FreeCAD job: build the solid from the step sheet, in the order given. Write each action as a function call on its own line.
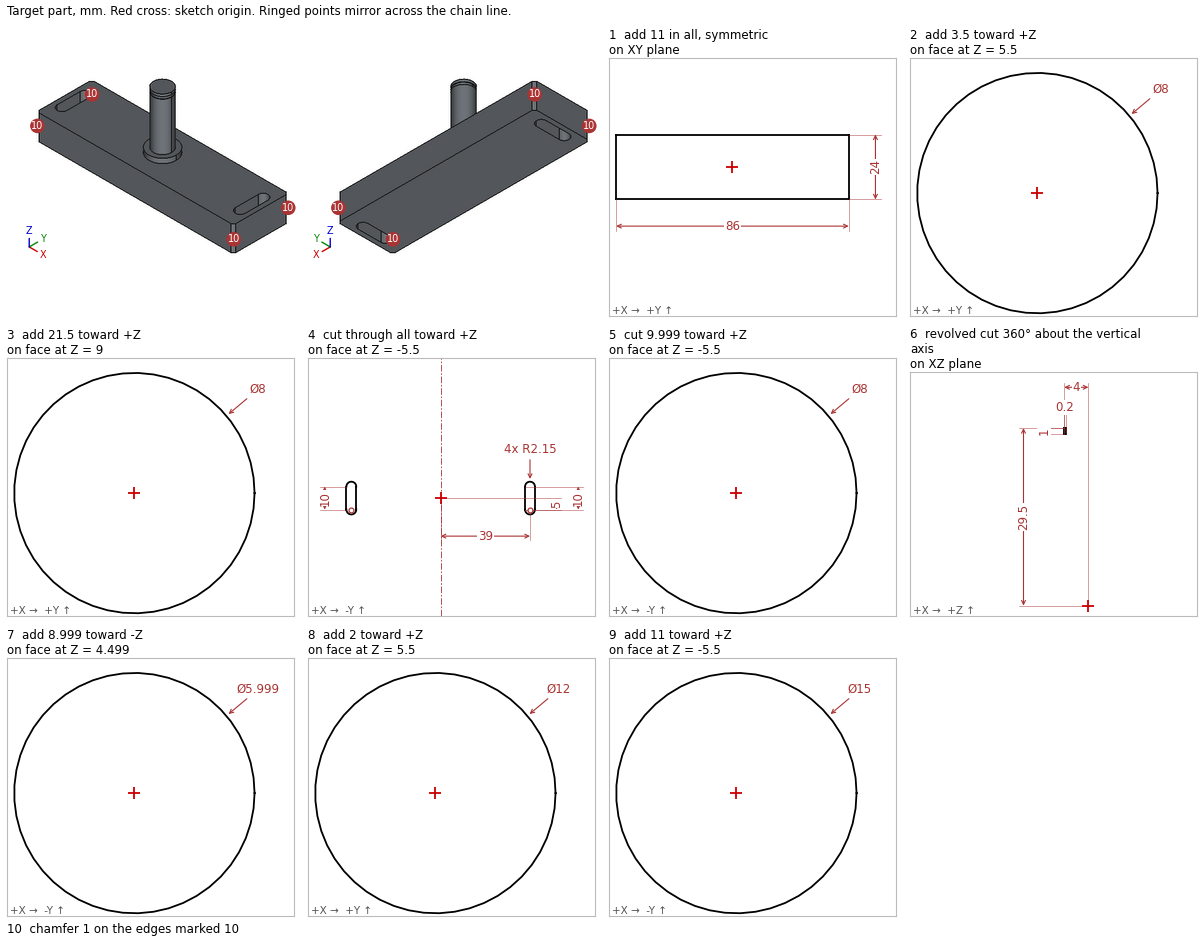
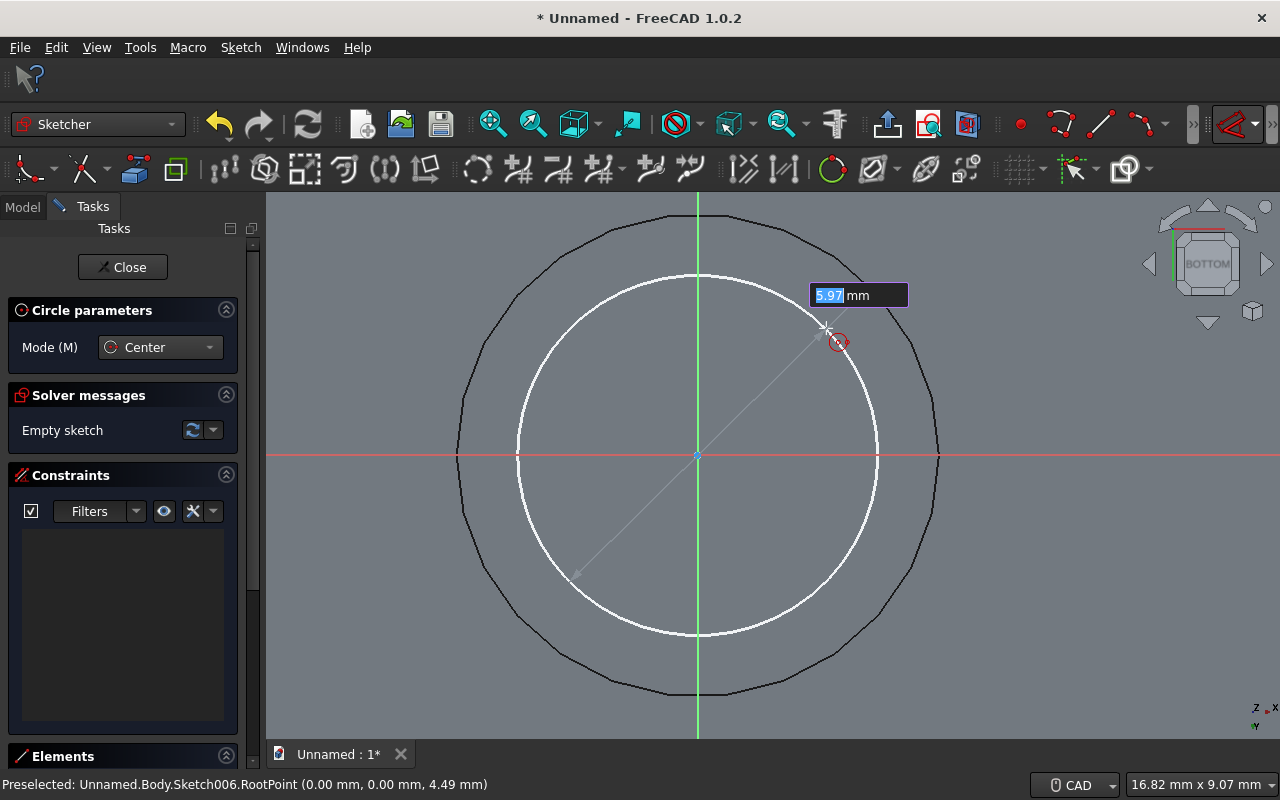
text(5.999)
key(Return)
key(Escape)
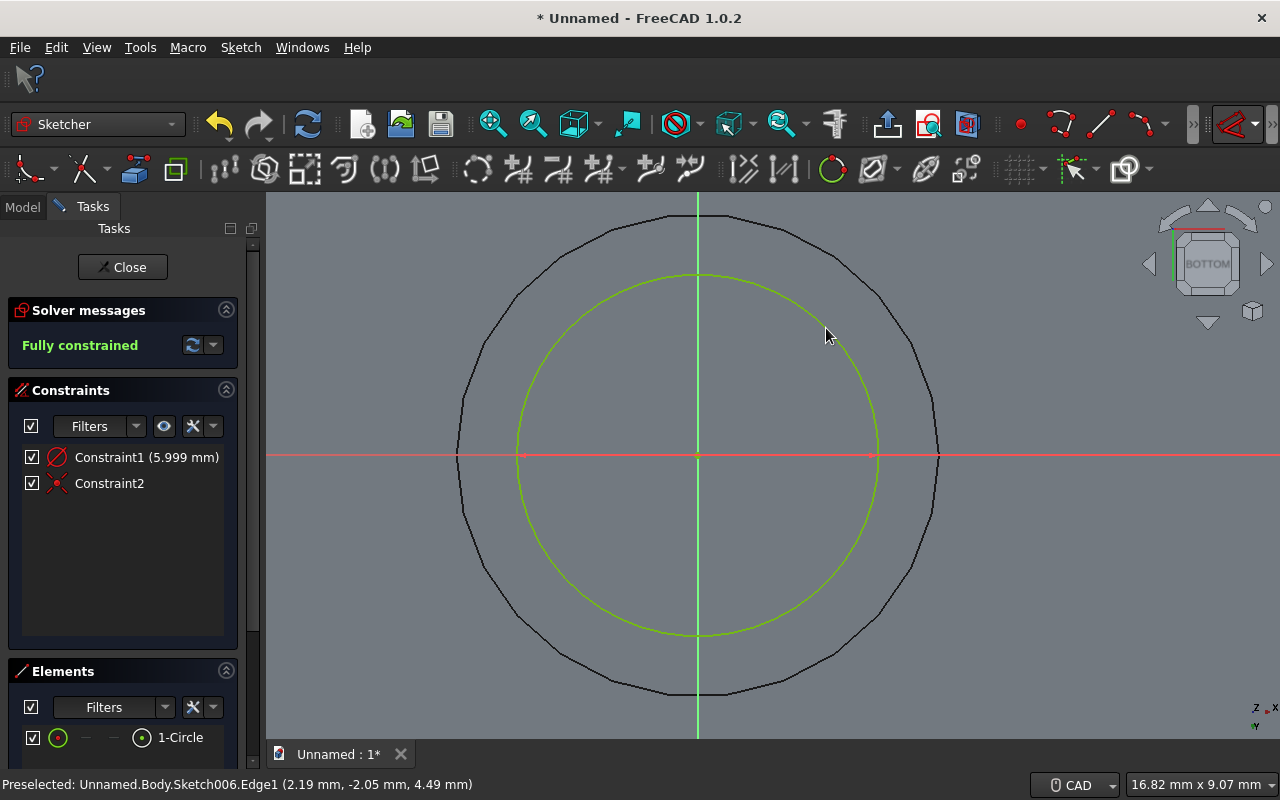
click(123, 267)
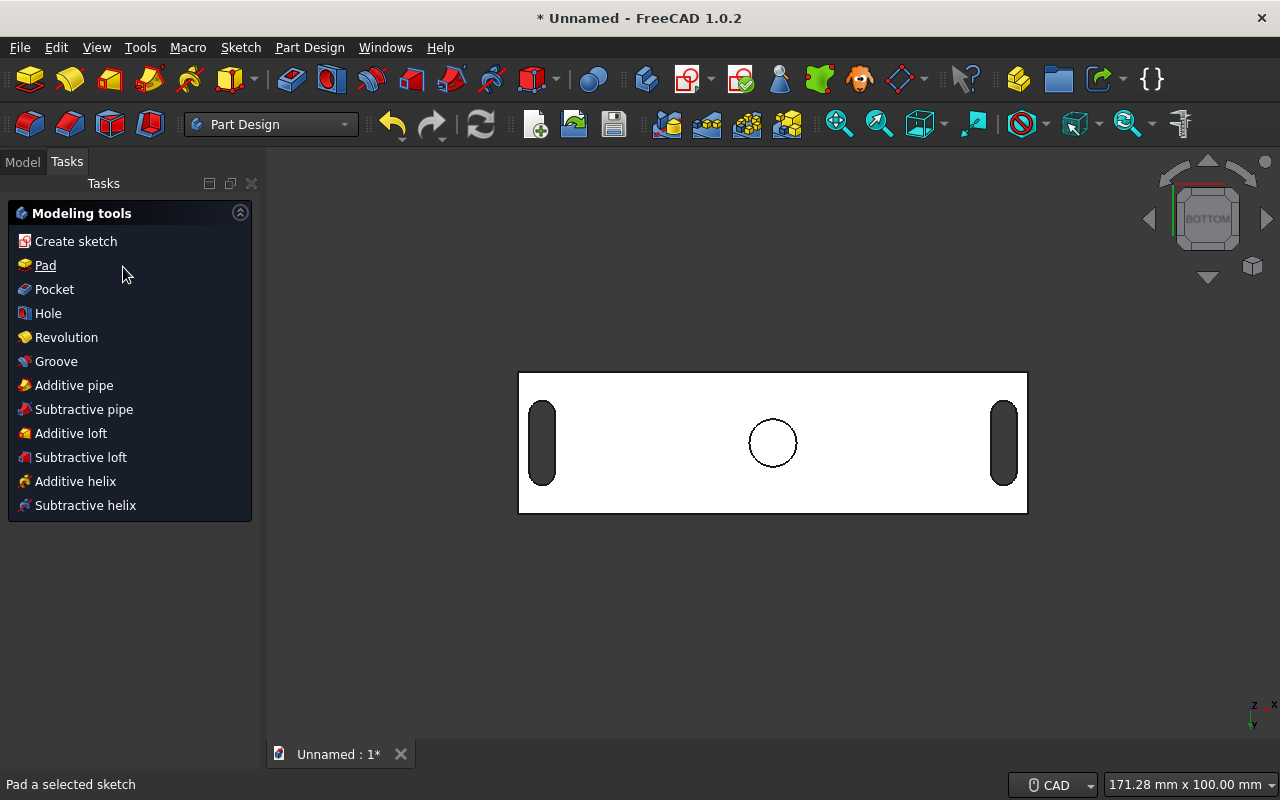
click(30, 80)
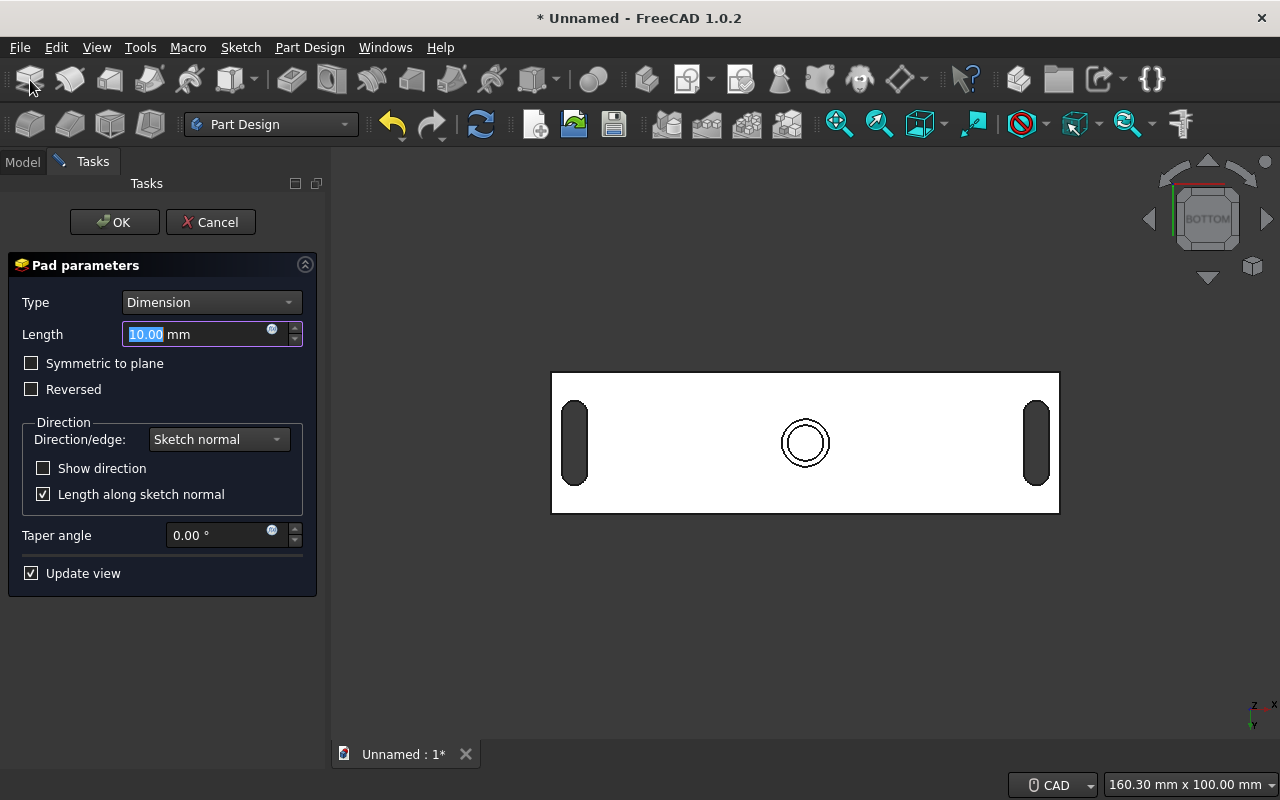
text(8.999)
key(Tab)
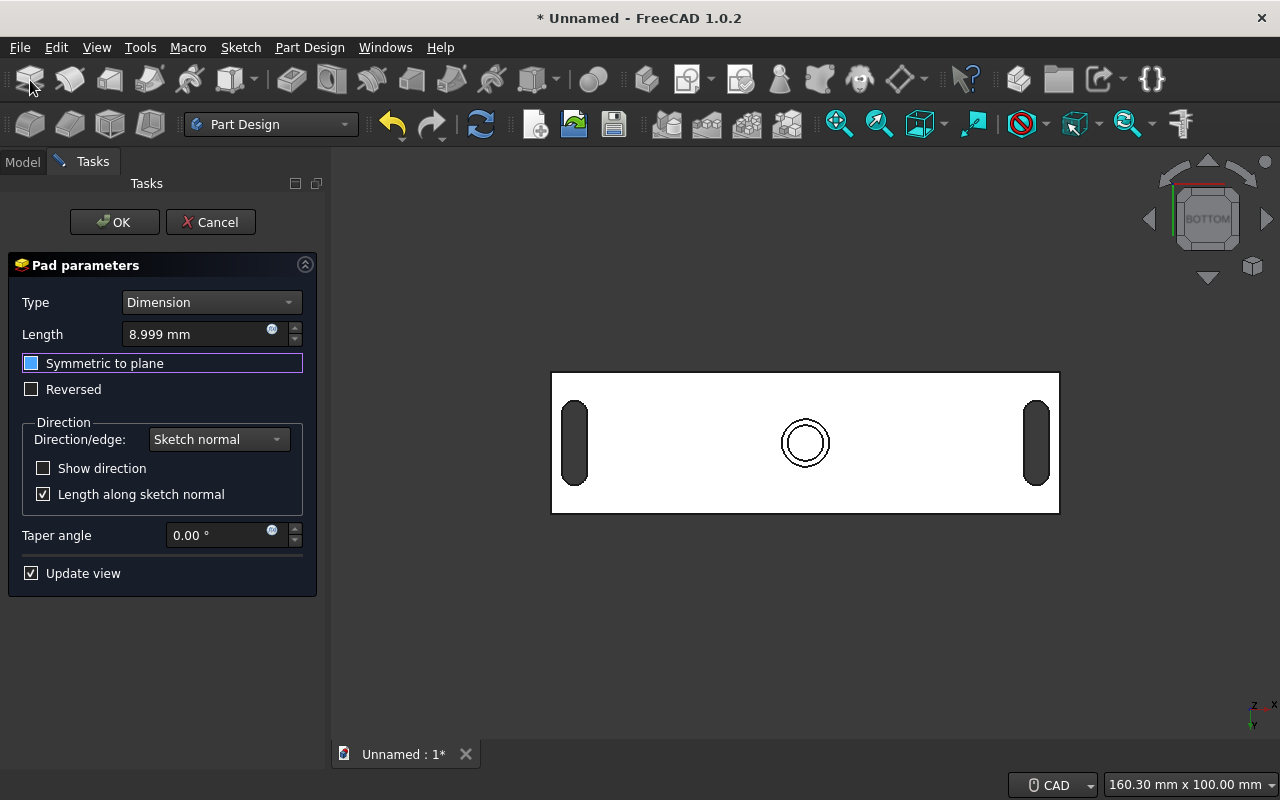
click(115, 222)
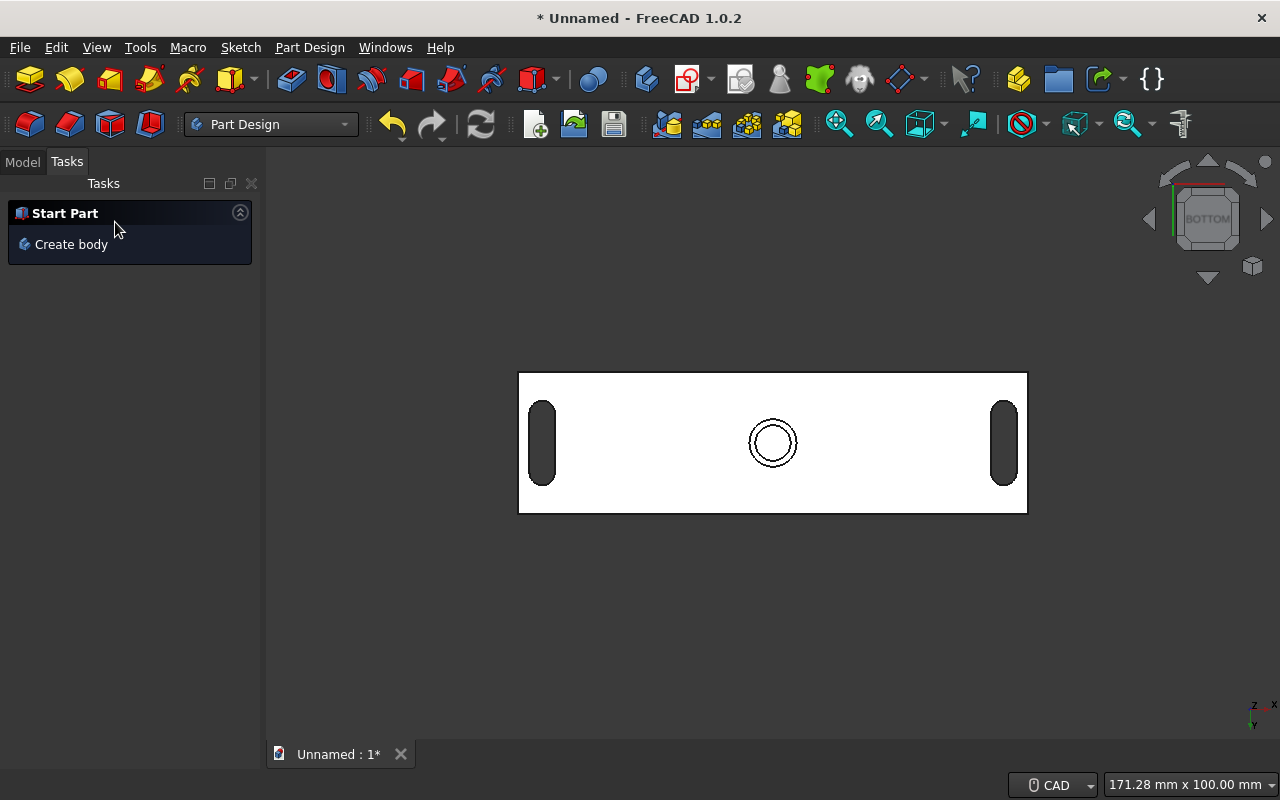
key(0)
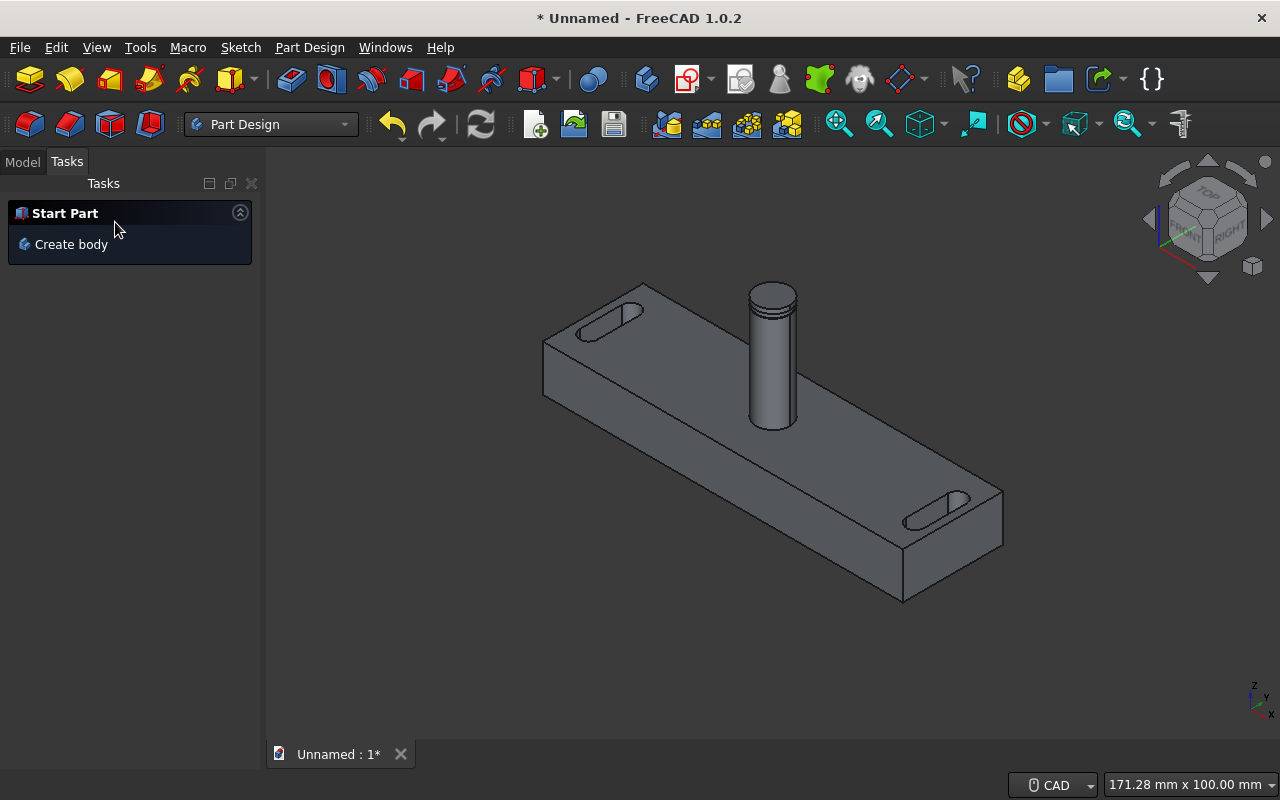
click(876, 475)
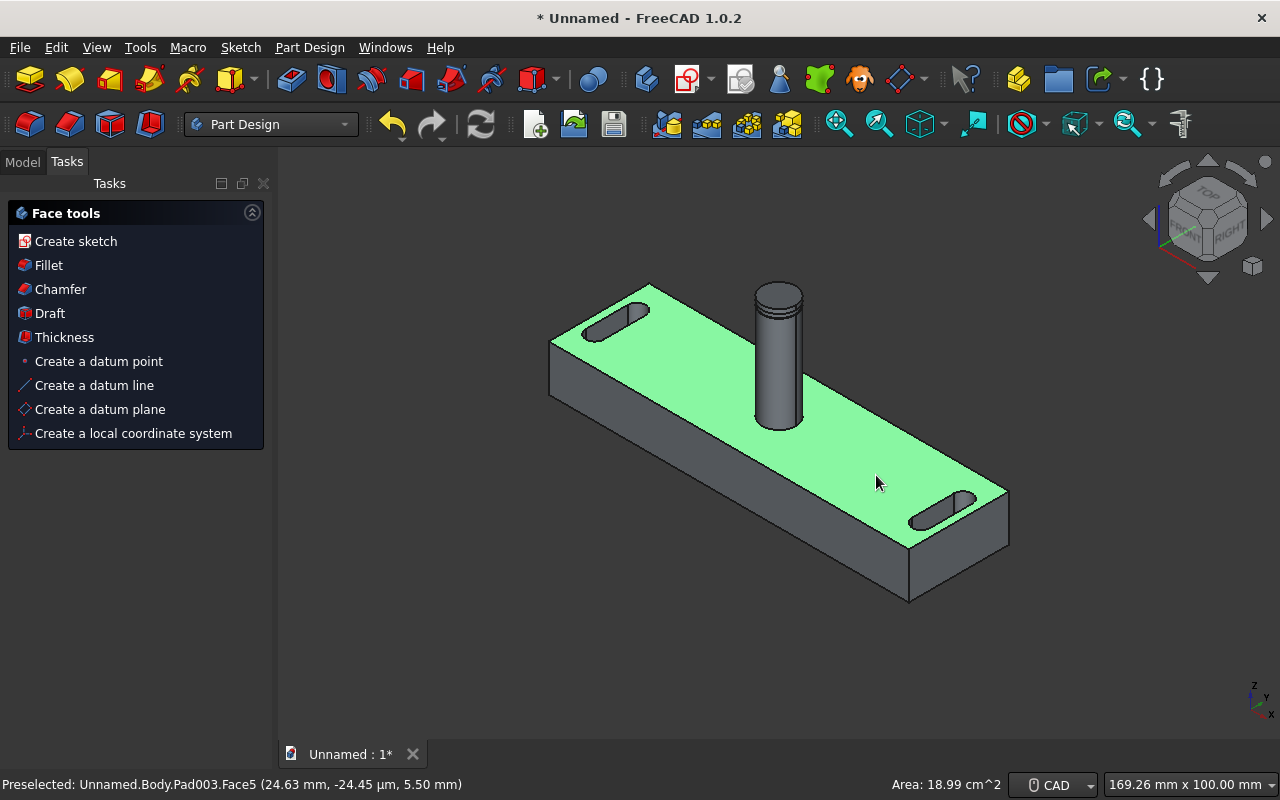
click(688, 80)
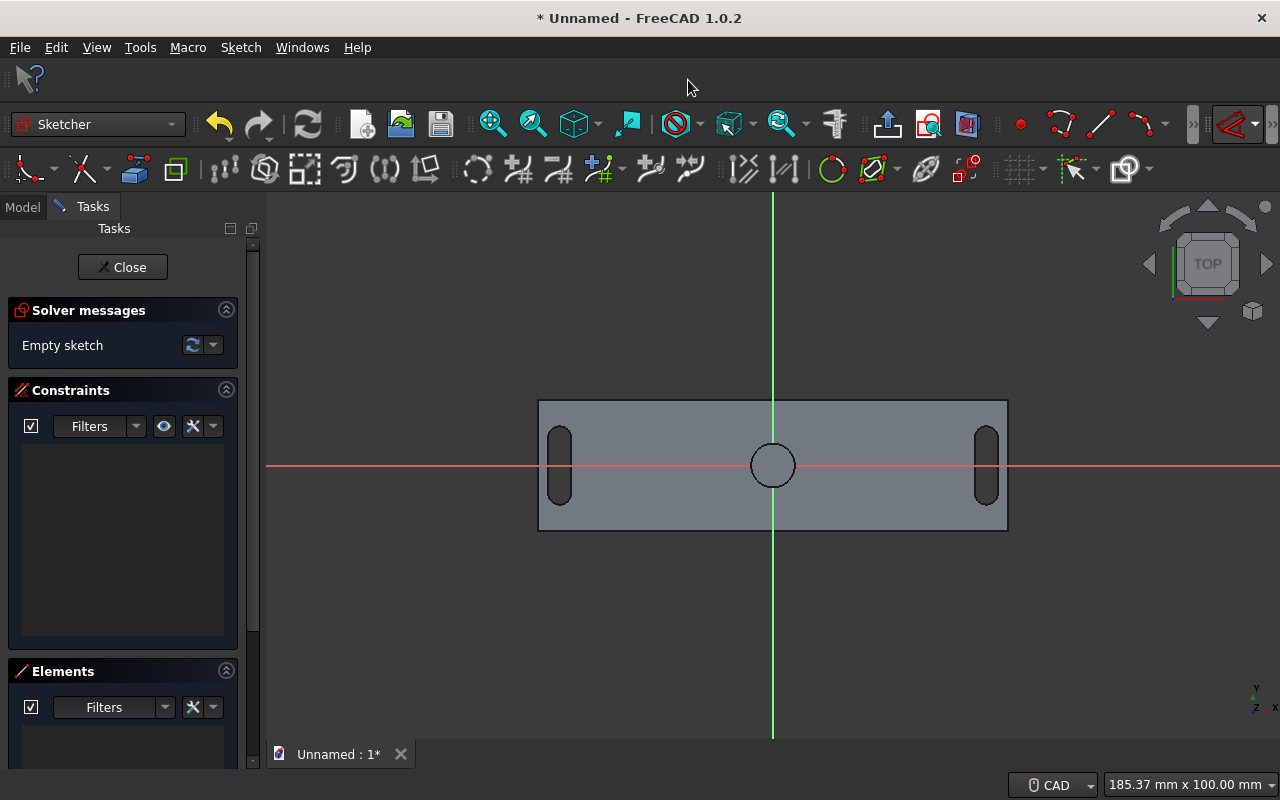
scroll(790, 465, up, 8)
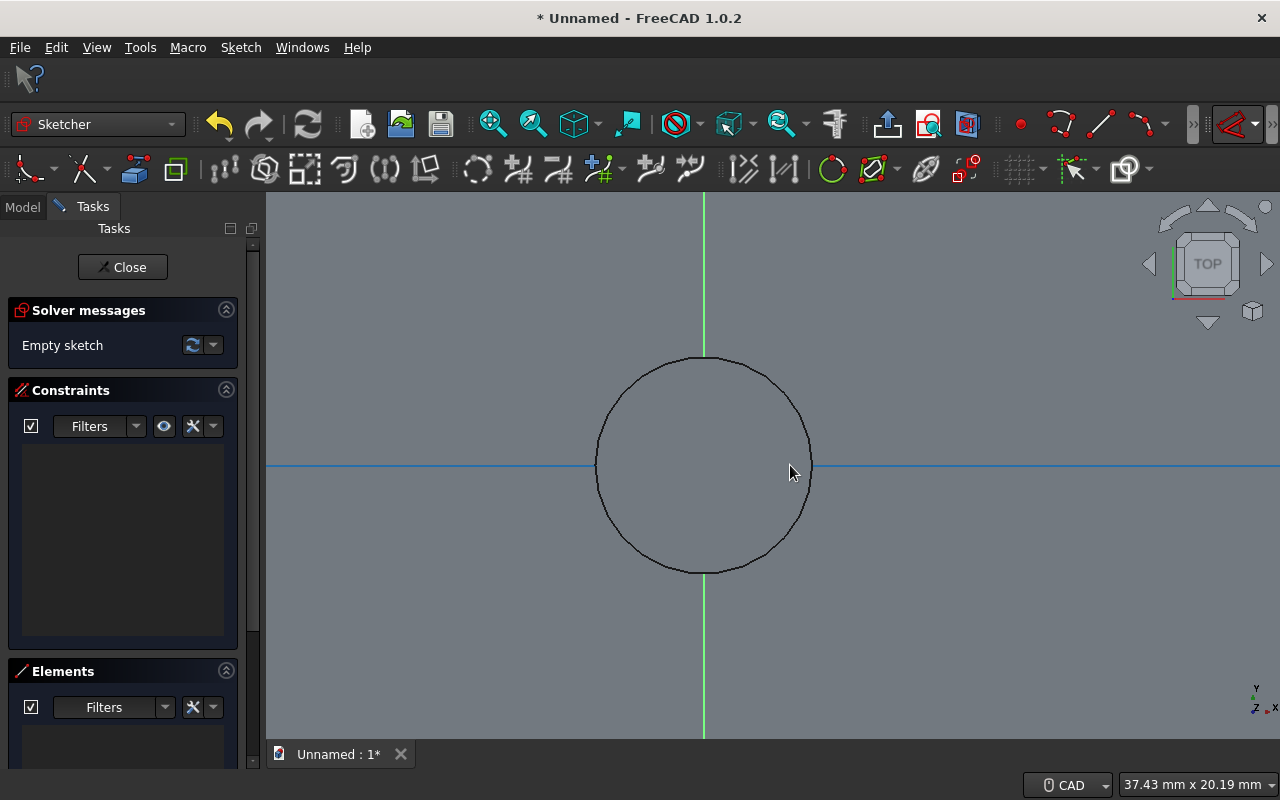
key(g)
key(c)